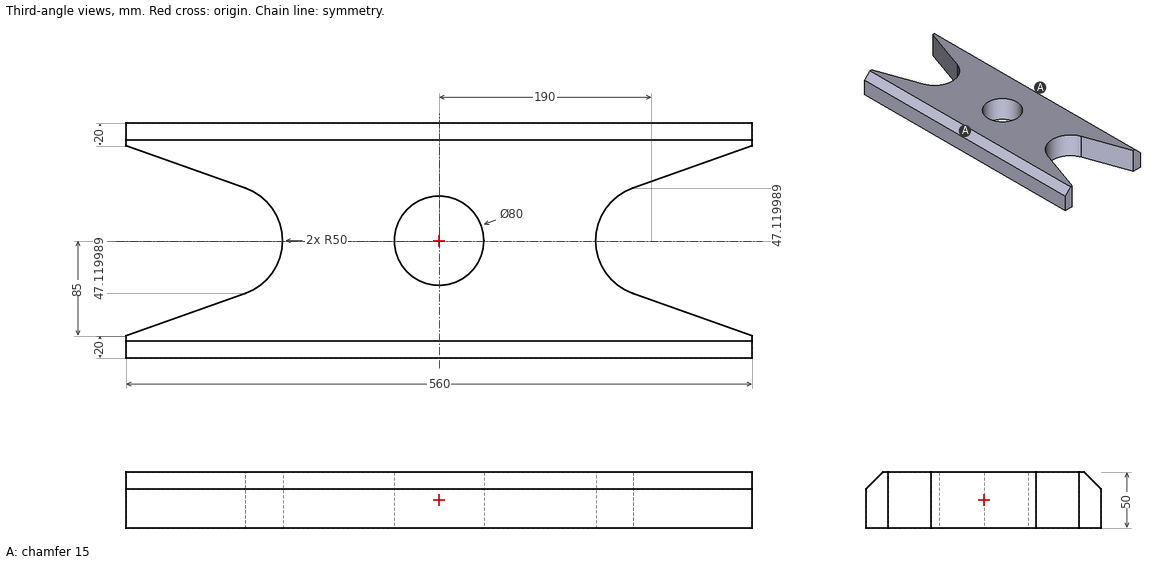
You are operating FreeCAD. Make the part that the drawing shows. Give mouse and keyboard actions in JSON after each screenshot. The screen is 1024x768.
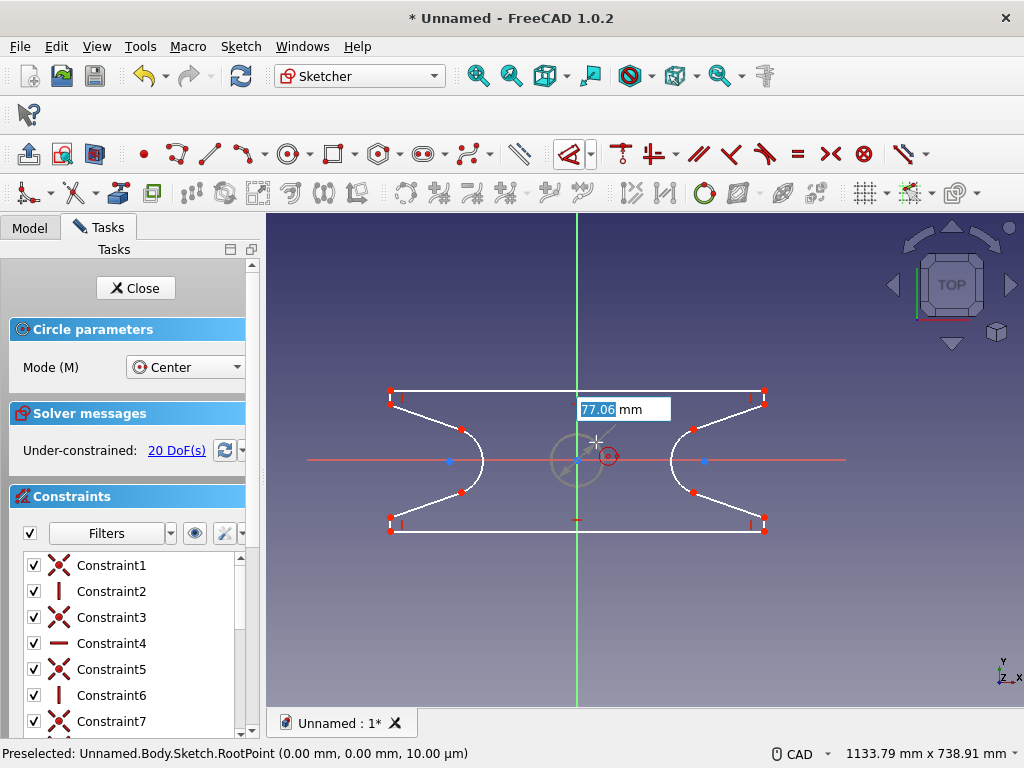
{"action": "type", "text": "80"}
{"action": "key", "text": "Return"}
{"action": "key", "text": "Escape"}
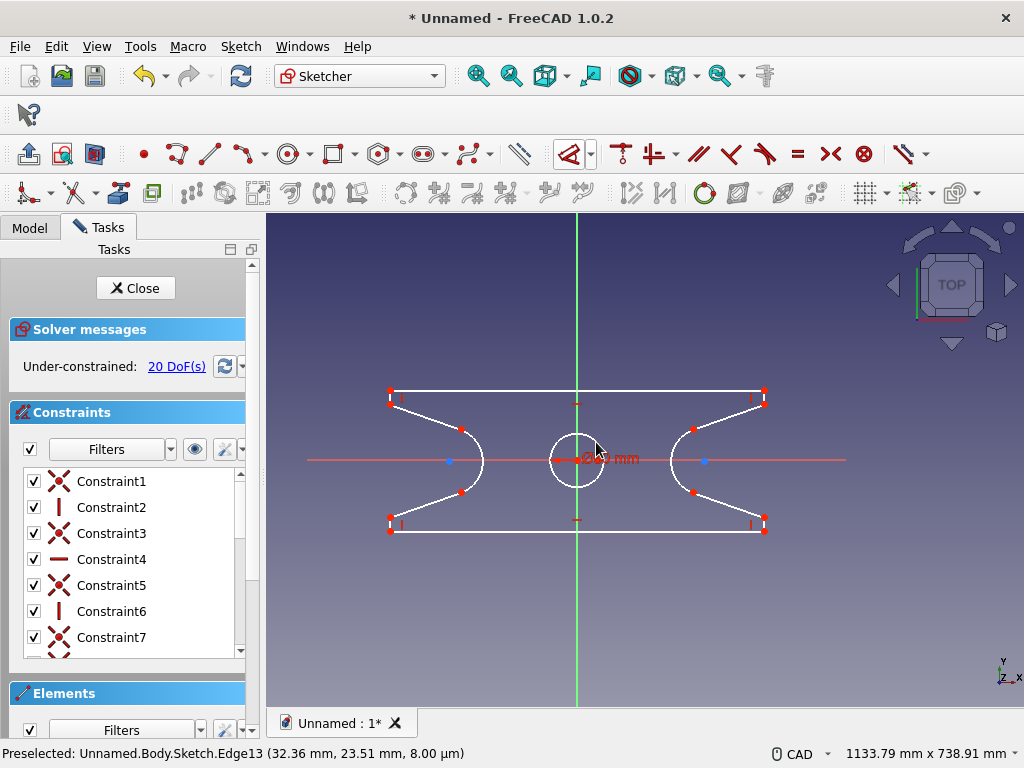
{"action": "left_click", "coordinate": [675, 446]}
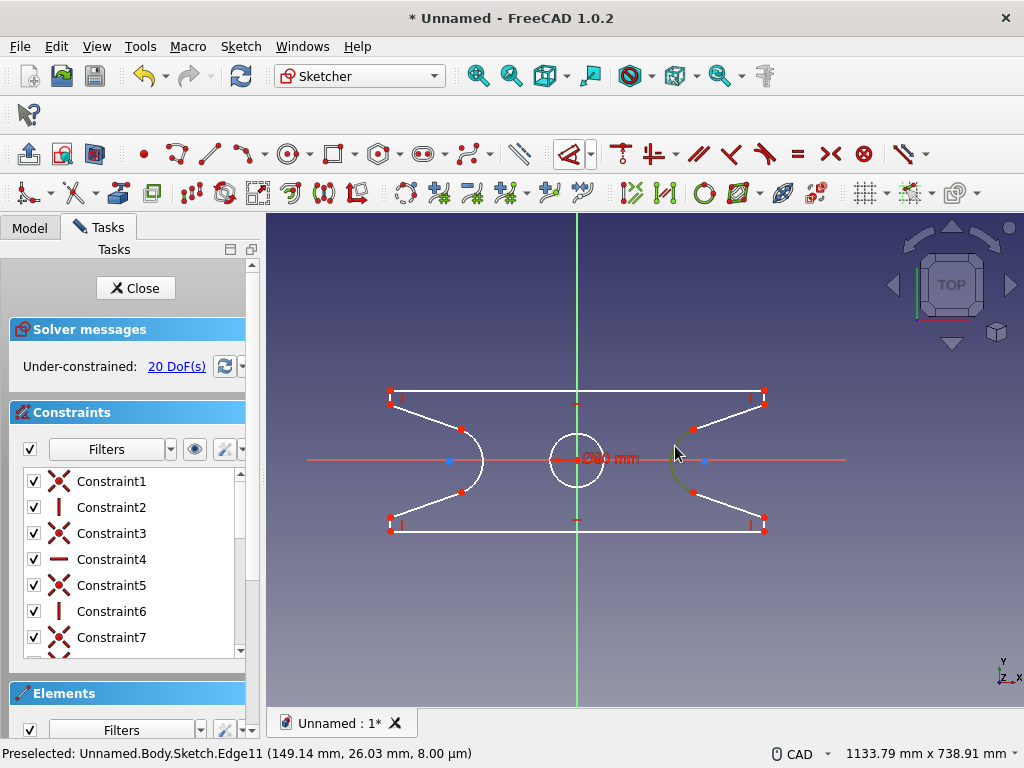
{"action": "left_click", "coordinate": [479, 477]}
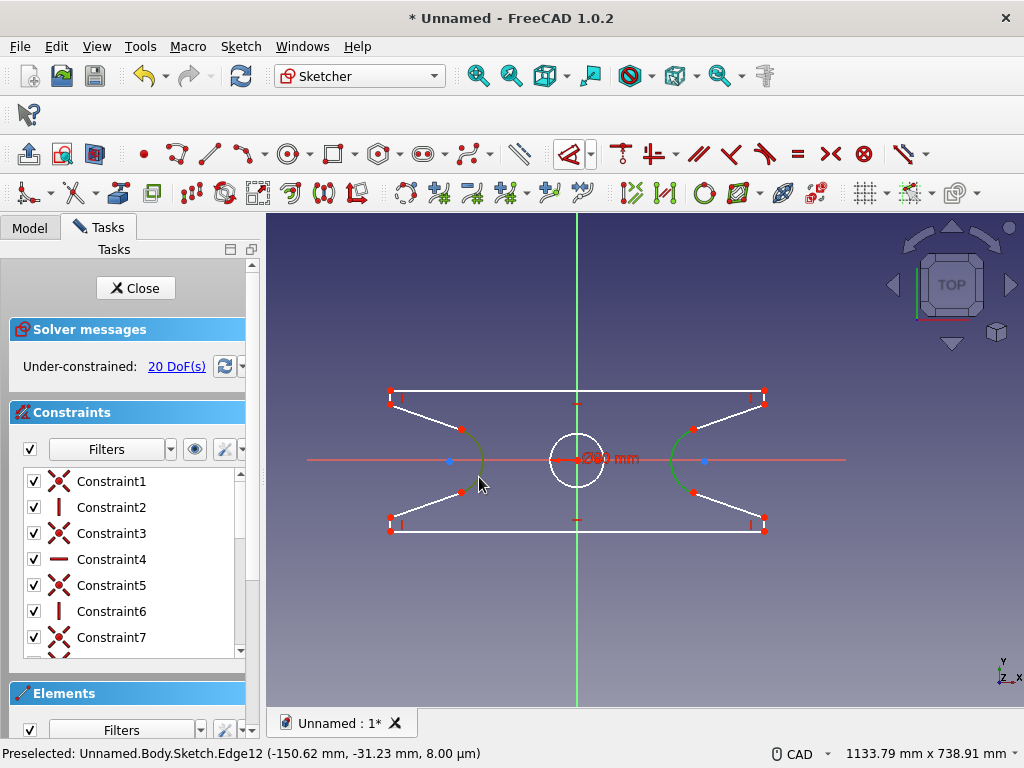
{"action": "key", "text": "e"}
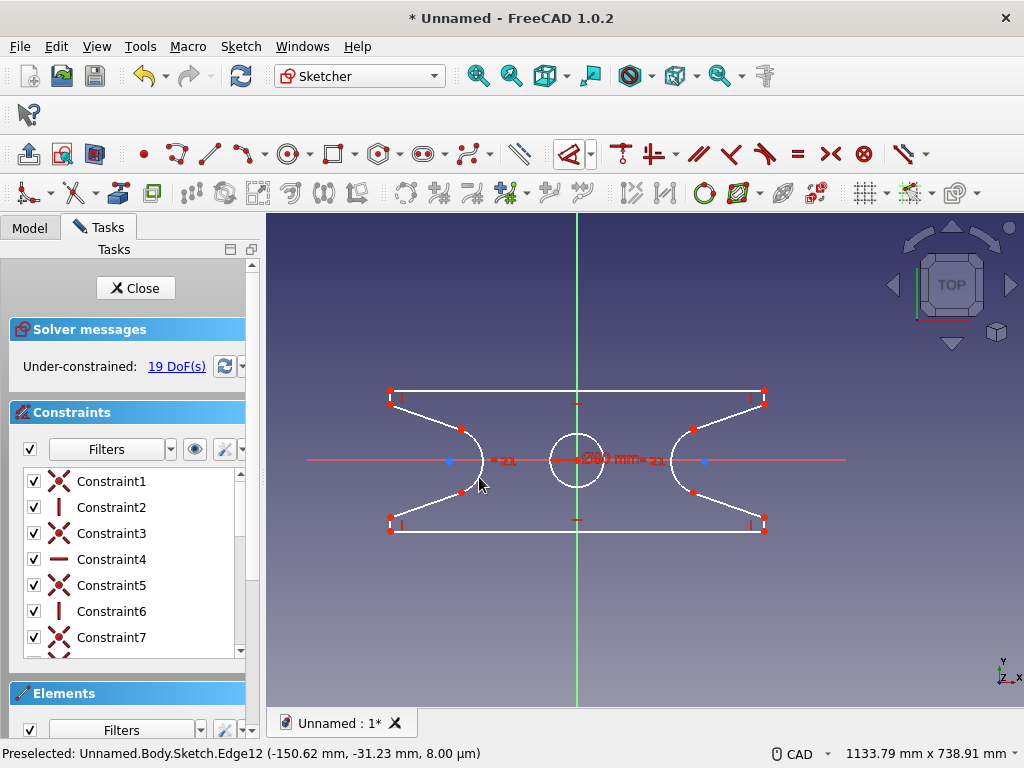
{"action": "left_click", "coordinate": [705, 462]}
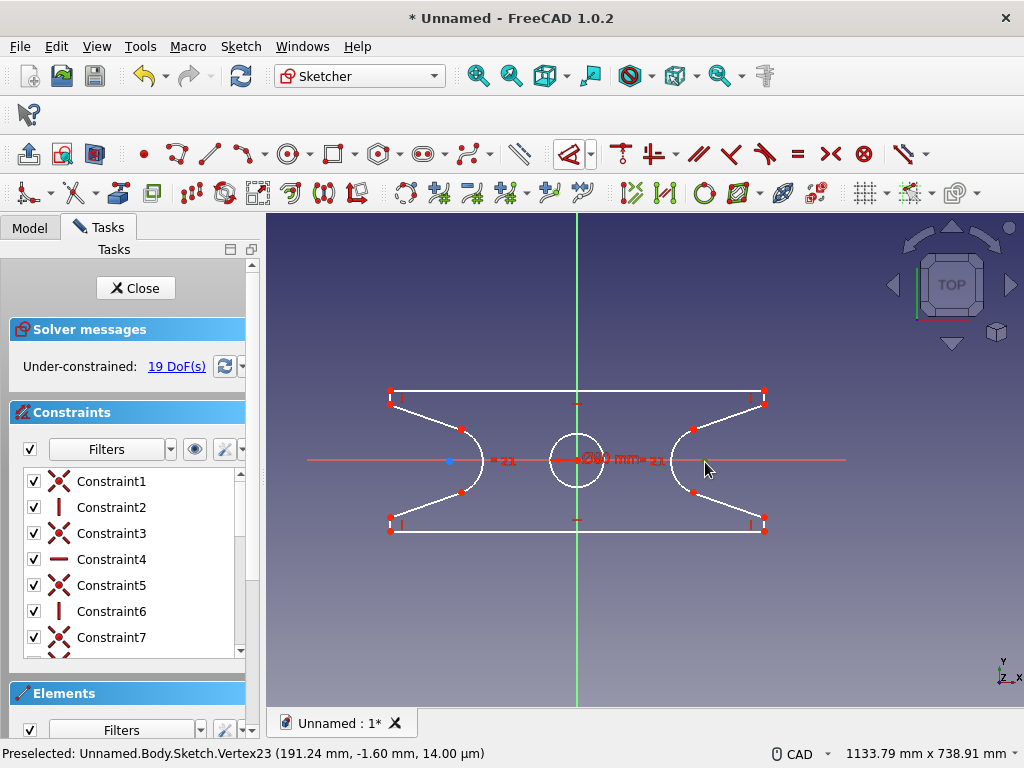
{"action": "left_click", "coordinate": [334, 460]}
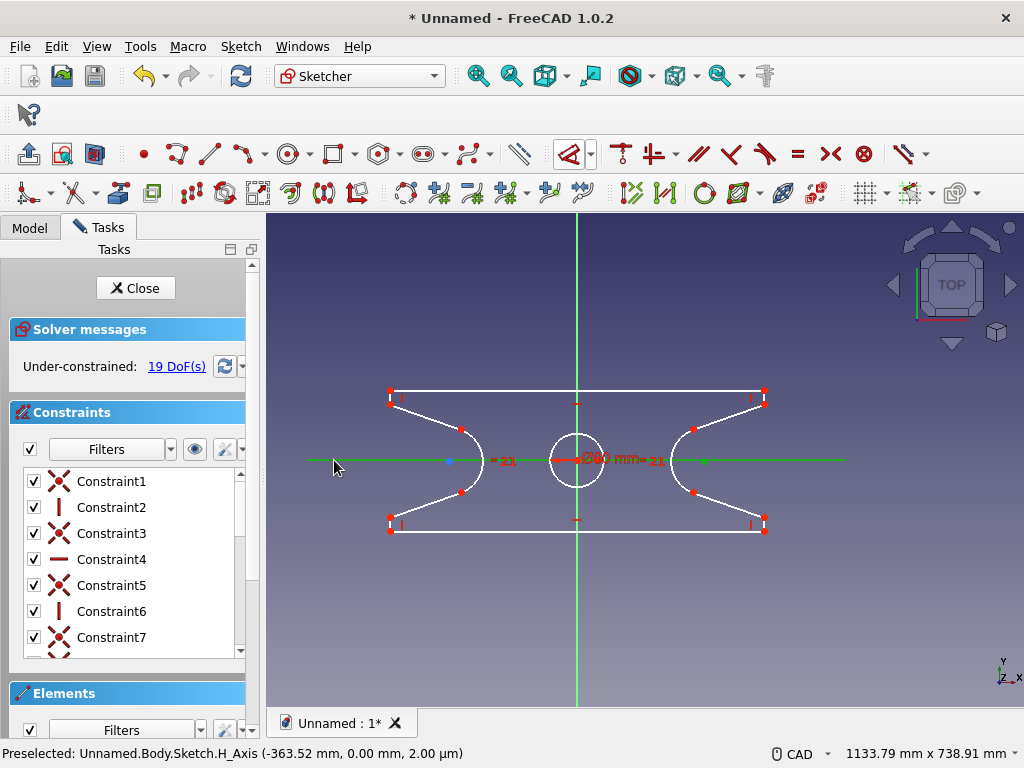
{"action": "left_click", "coordinate": [621, 154]}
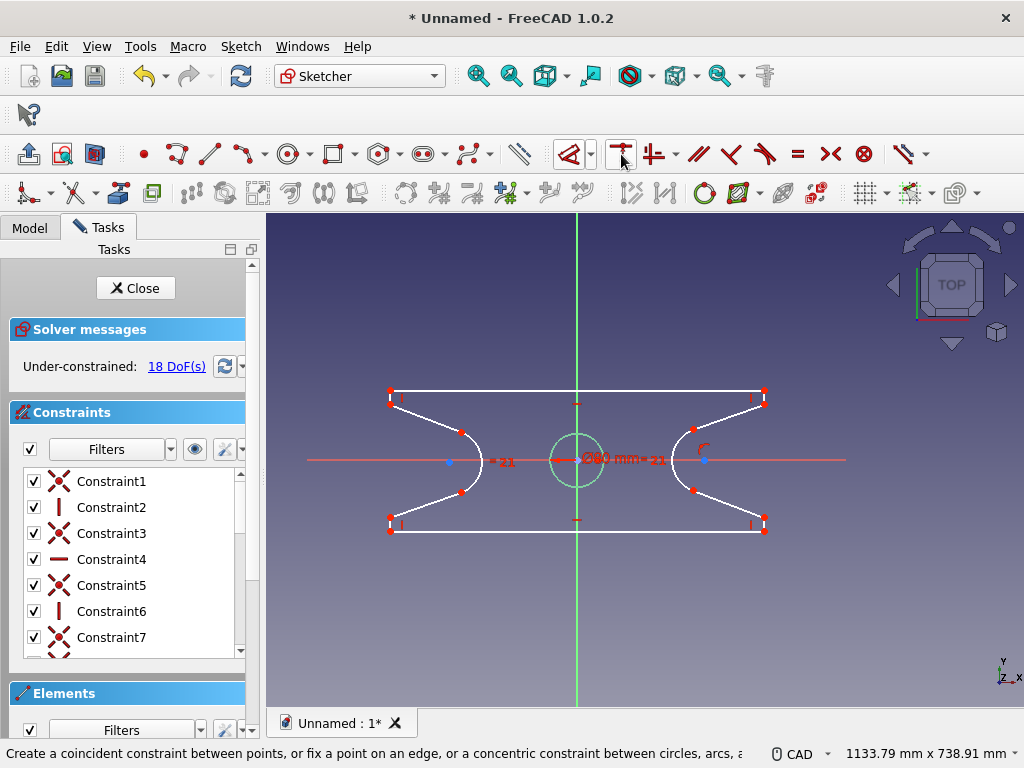
{"action": "left_click", "coordinate": [449, 463]}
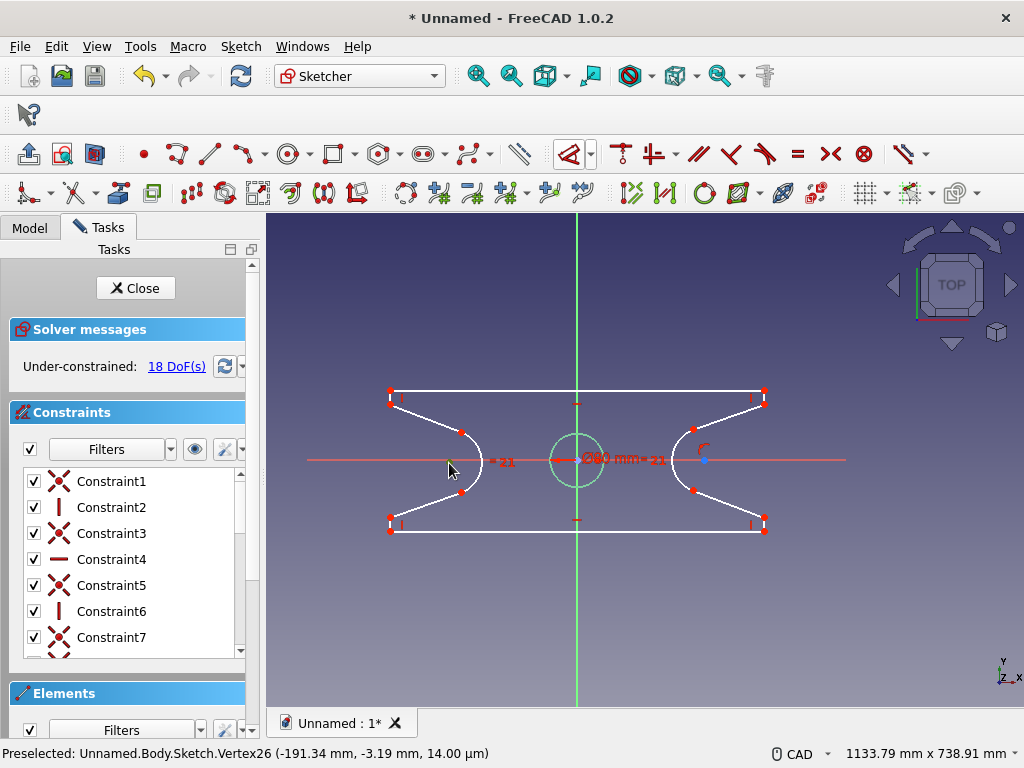
{"action": "left_click", "coordinate": [334, 460]}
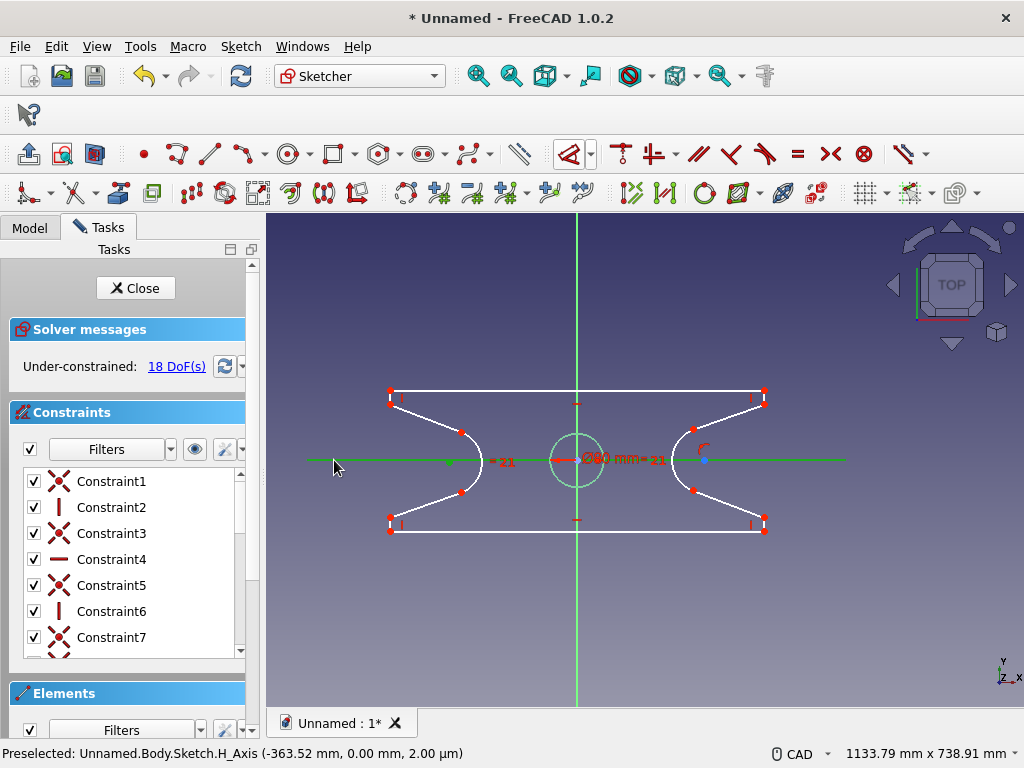
{"action": "key", "text": "c"}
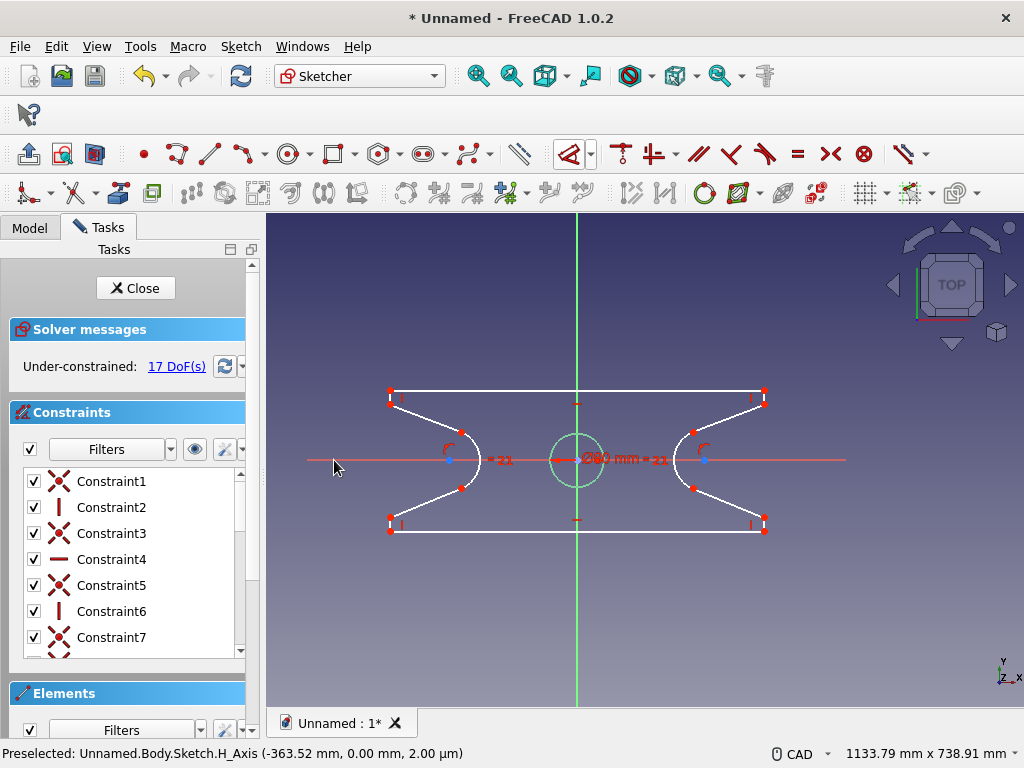
{"action": "left_click", "coordinate": [390, 518]}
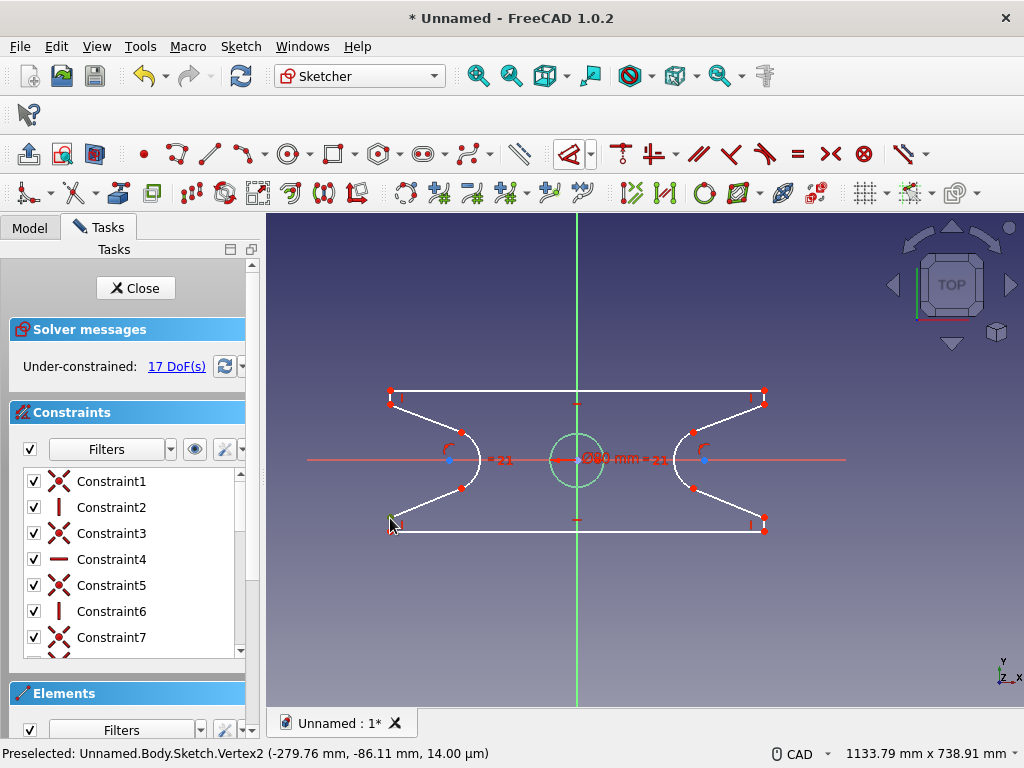
{"action": "left_click", "coordinate": [764, 518]}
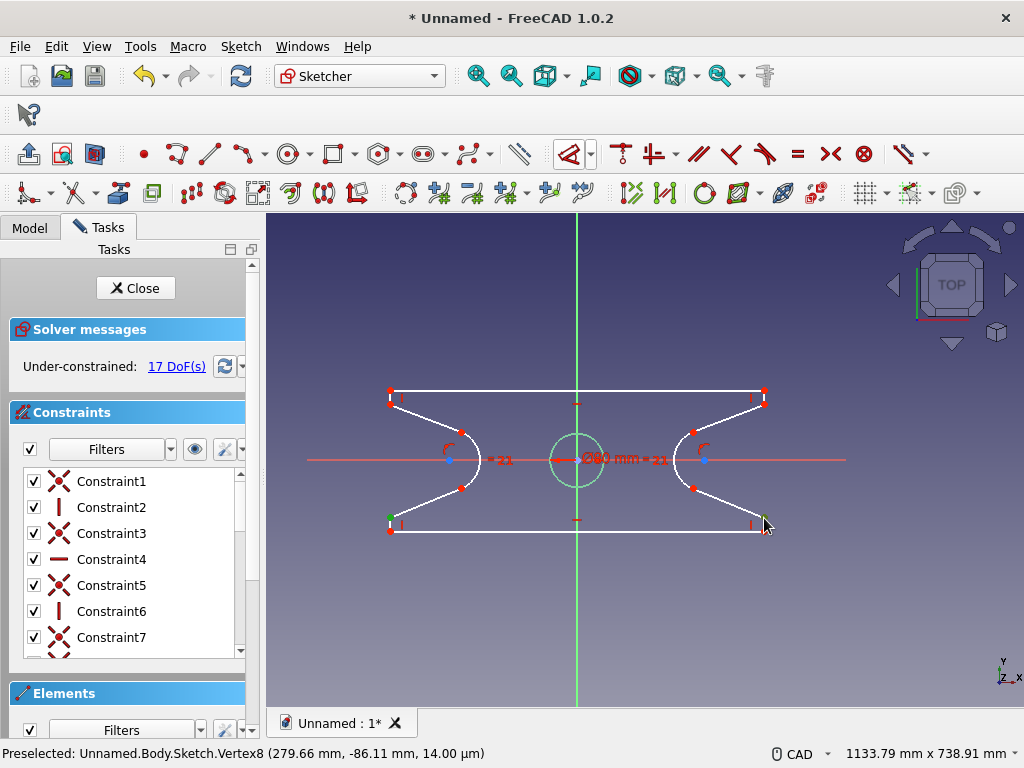
{"action": "left_click", "coordinate": [577, 648]}